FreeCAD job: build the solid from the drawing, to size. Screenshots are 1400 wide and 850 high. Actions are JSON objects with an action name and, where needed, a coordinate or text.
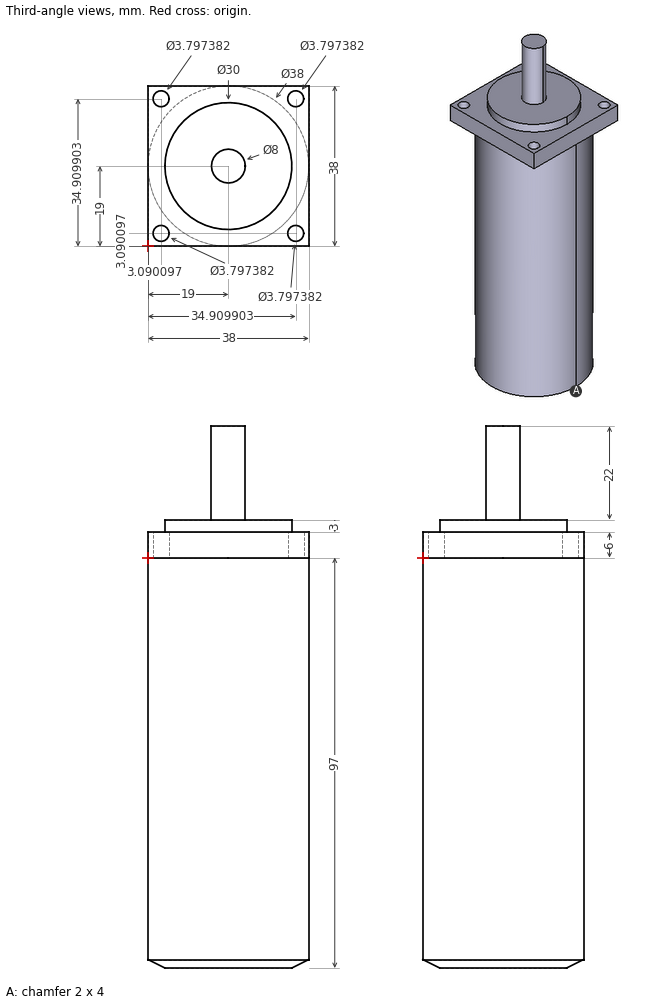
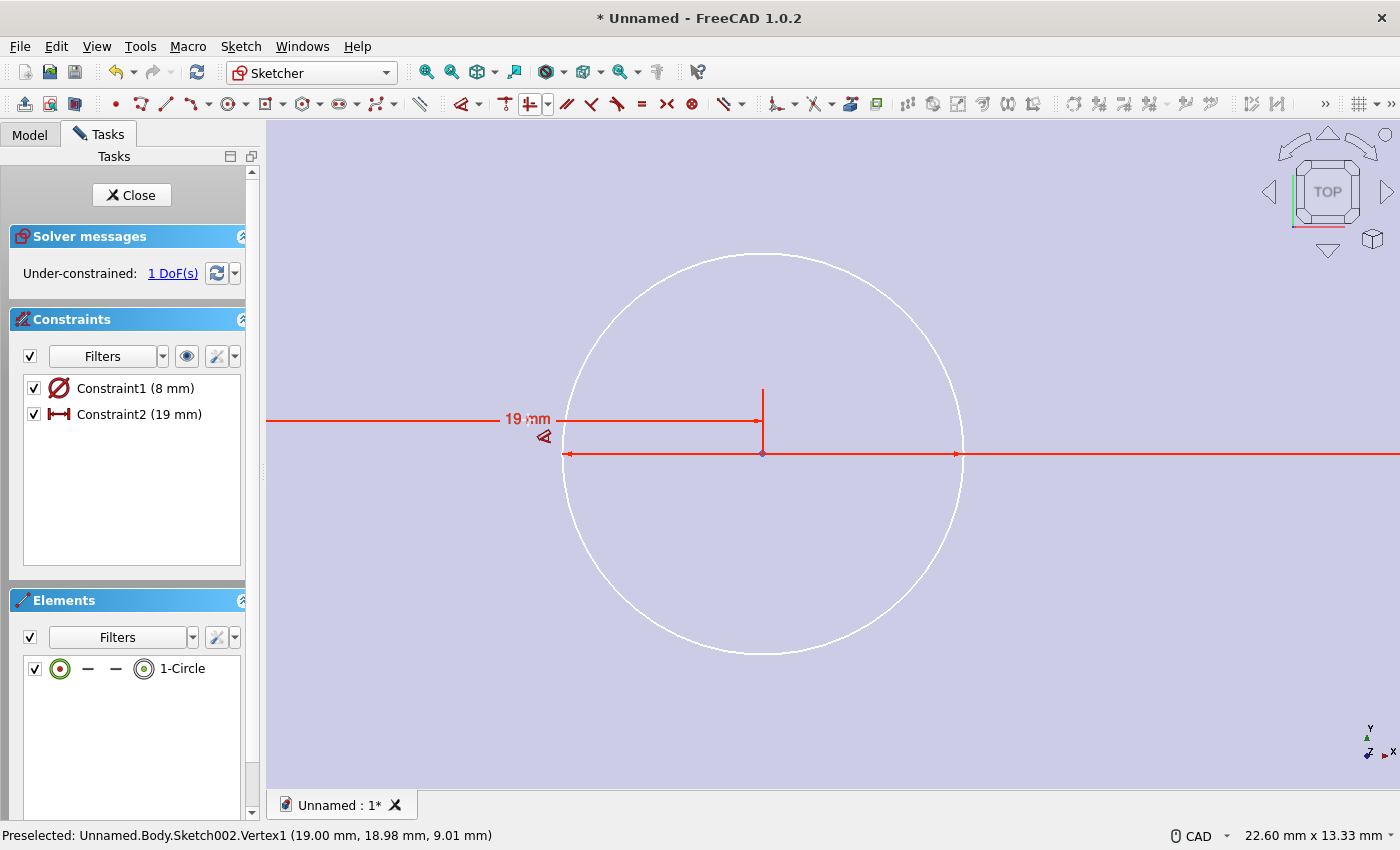
{"action": "left_click", "coordinate": [763, 454]}
{"action": "left_click", "coordinate": [797, 608]}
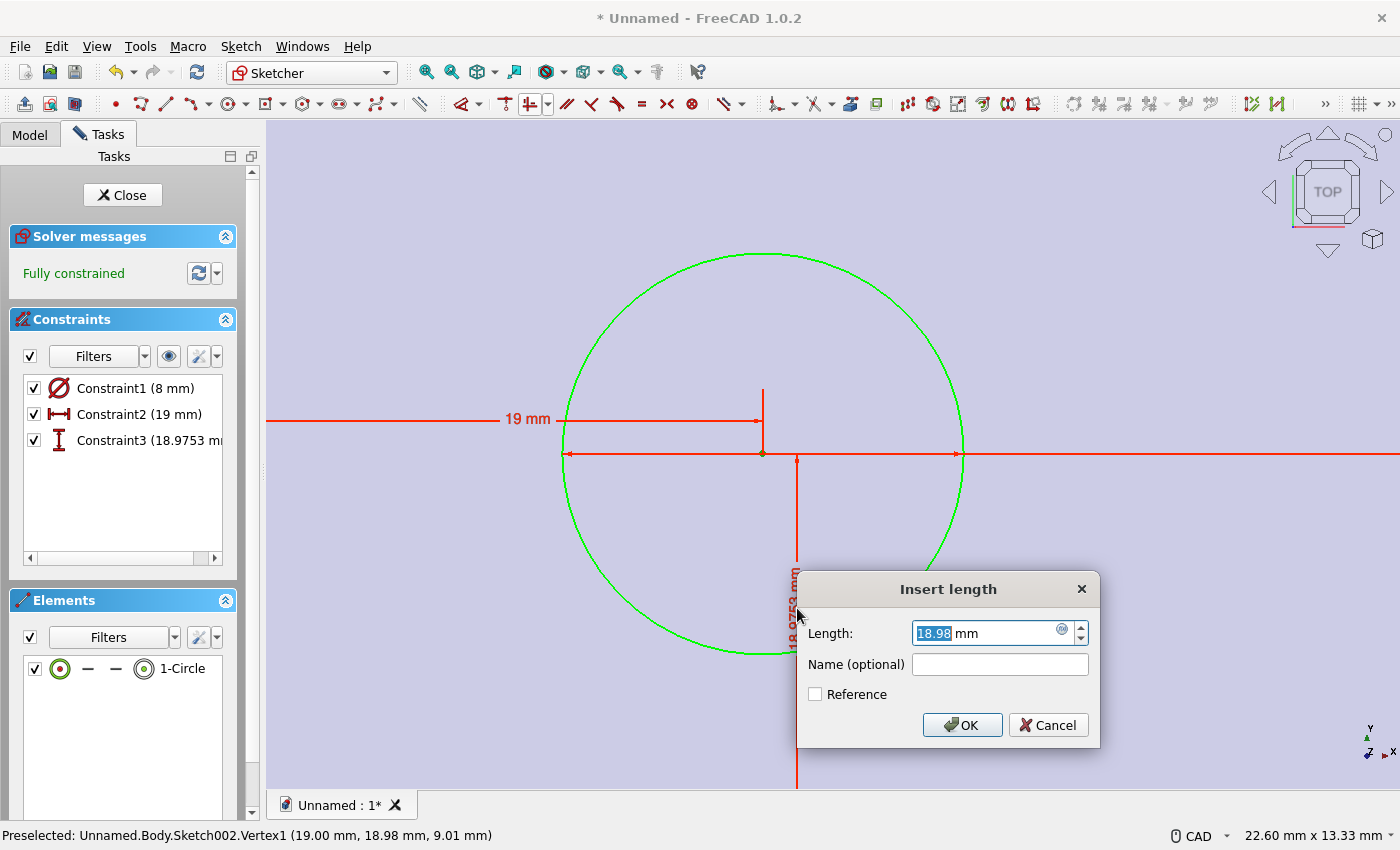
{"action": "type", "text": "19"}
{"action": "key", "text": "Return"}
{"action": "key", "text": "Escape"}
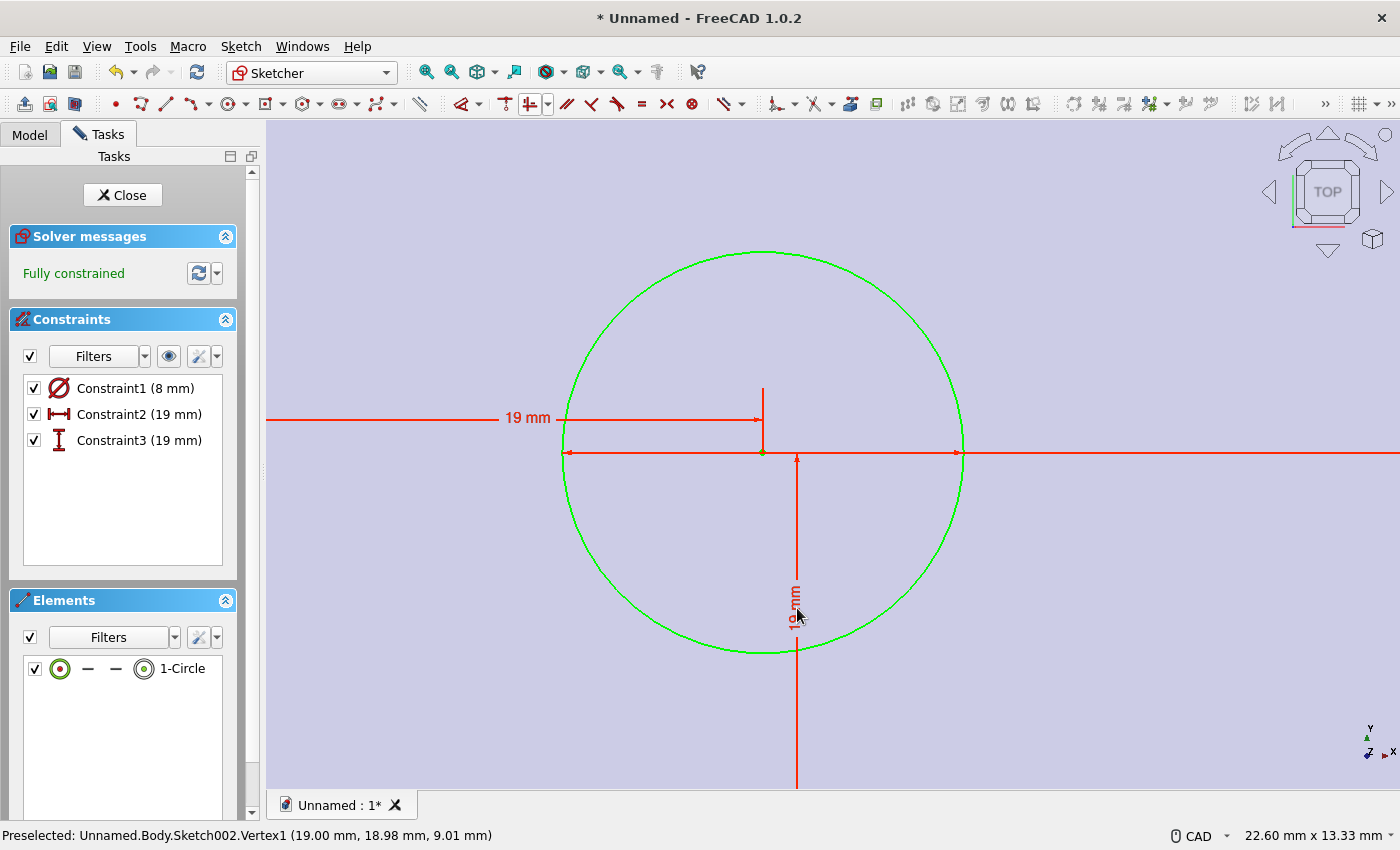
{"action": "left_click", "coordinate": [123, 195]}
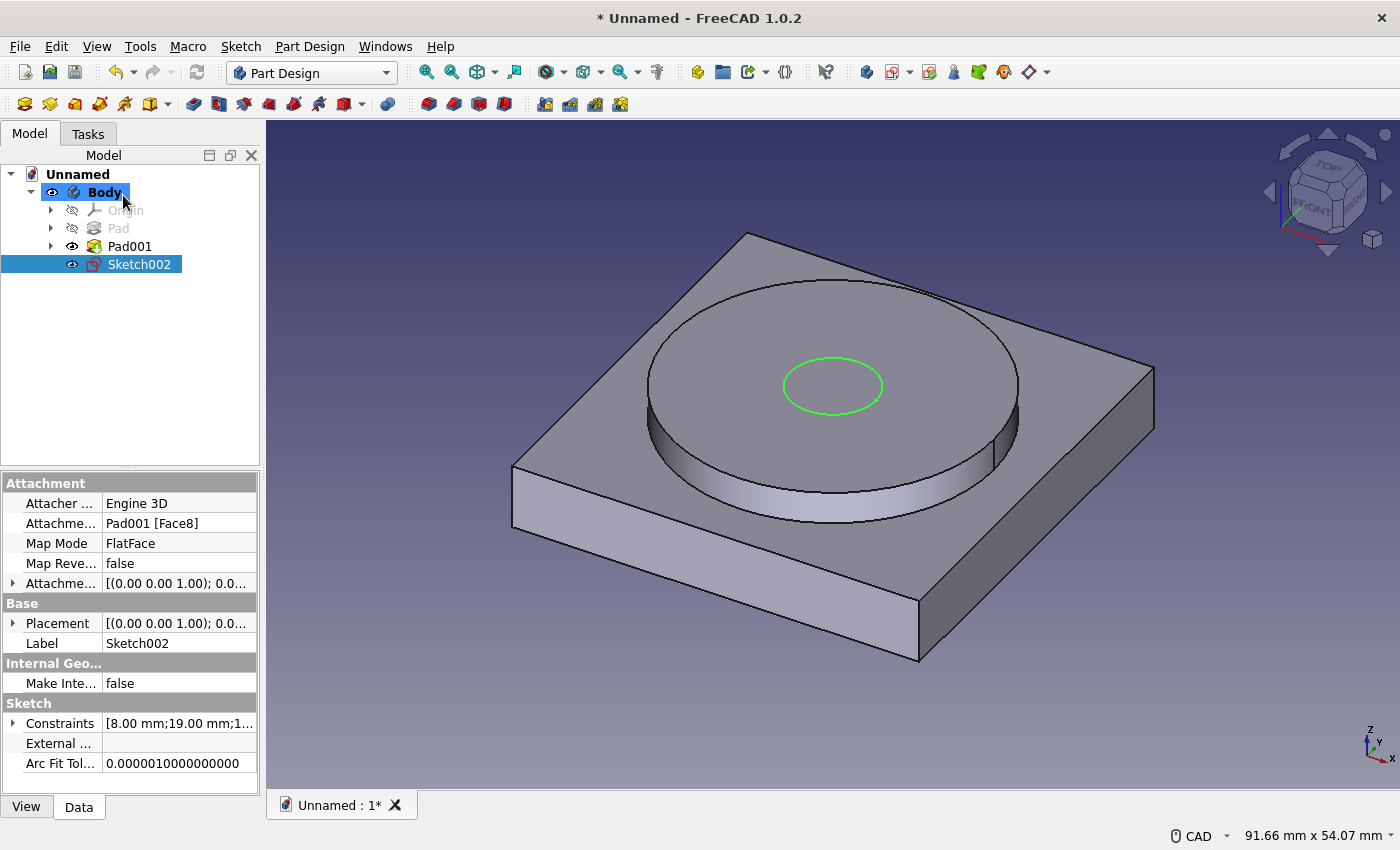
{"action": "left_click", "coordinate": [25, 104]}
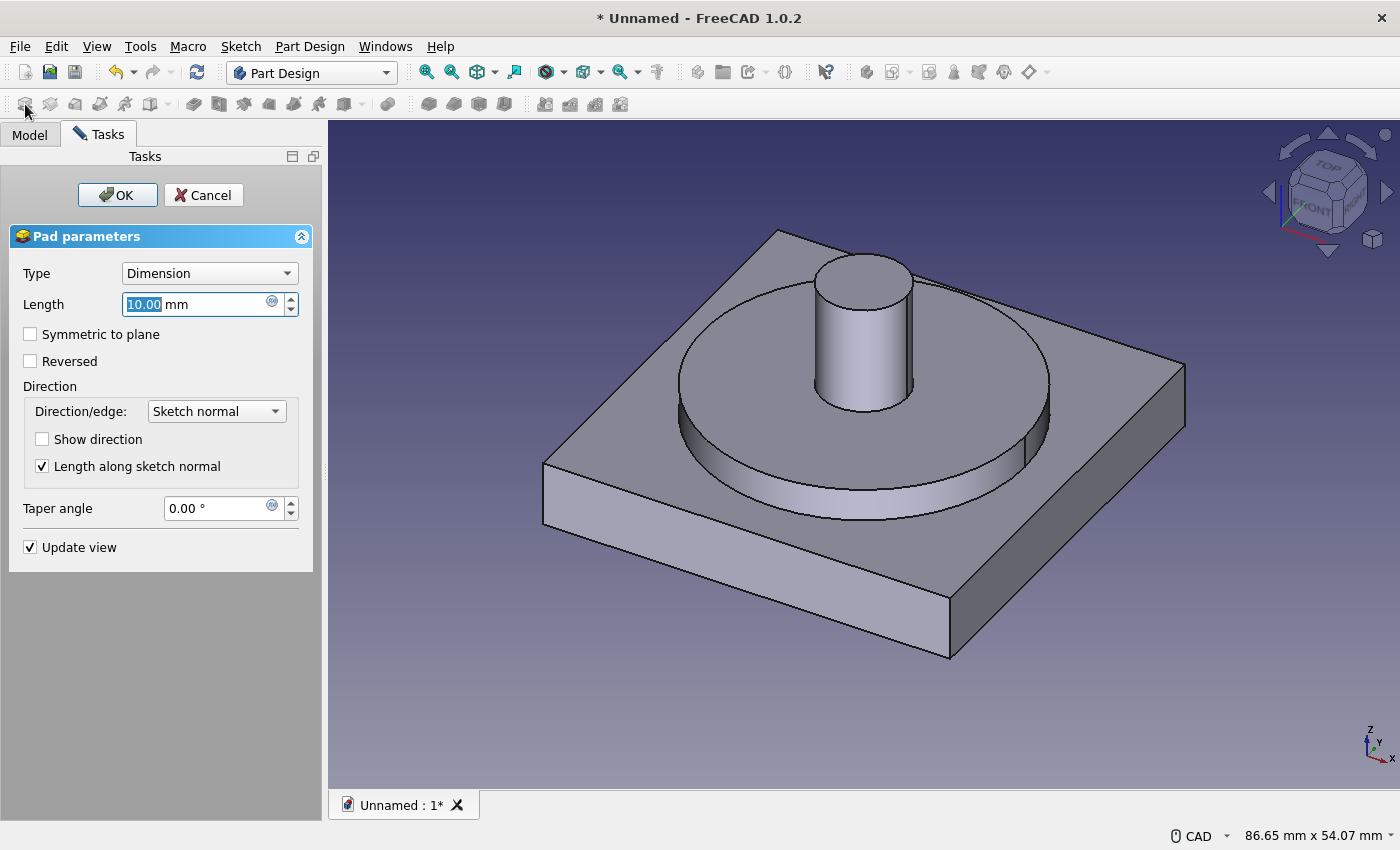
{"action": "type", "text": "22"}
{"action": "key", "text": "Tab"}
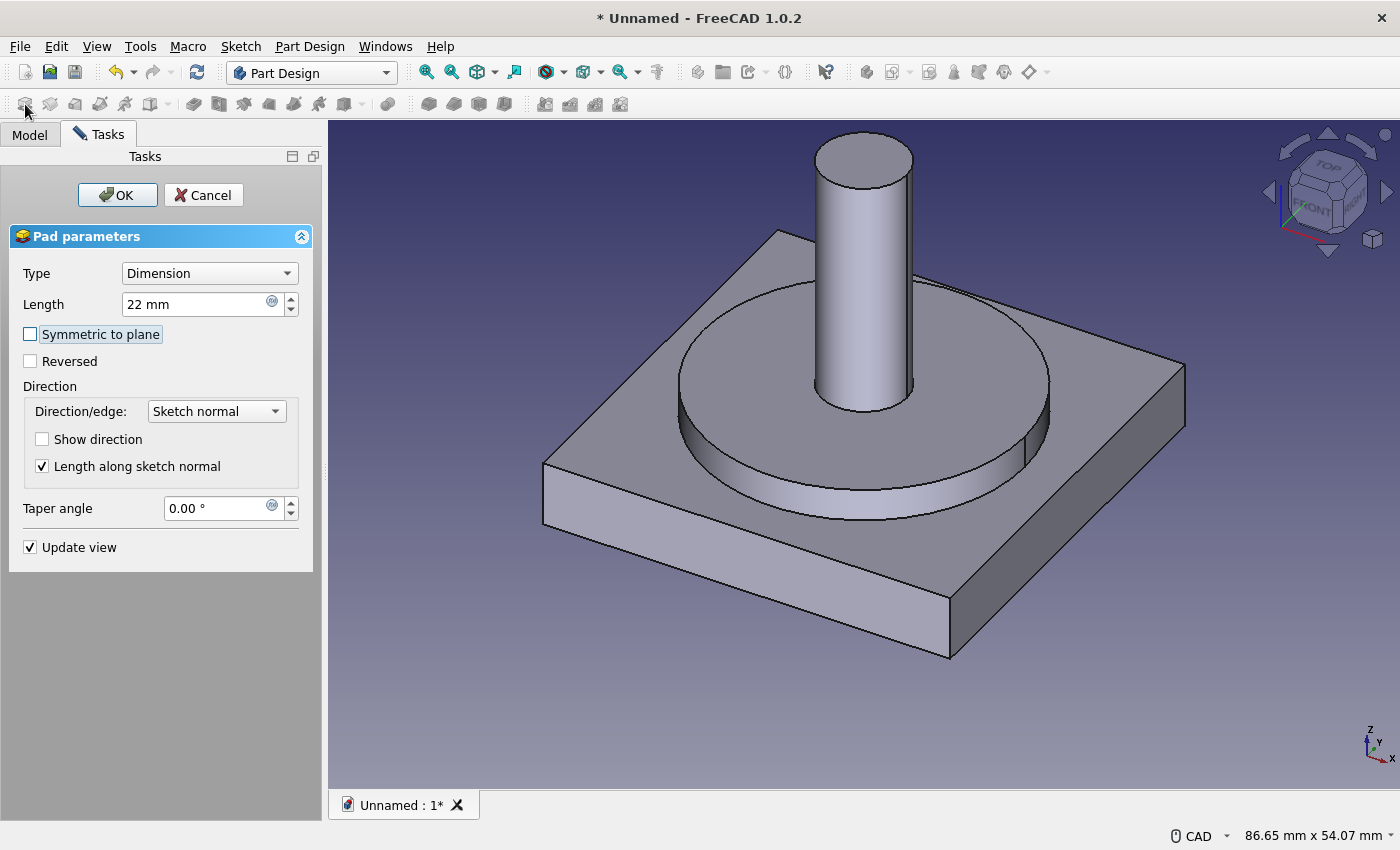
{"action": "left_click", "coordinate": [118, 195]}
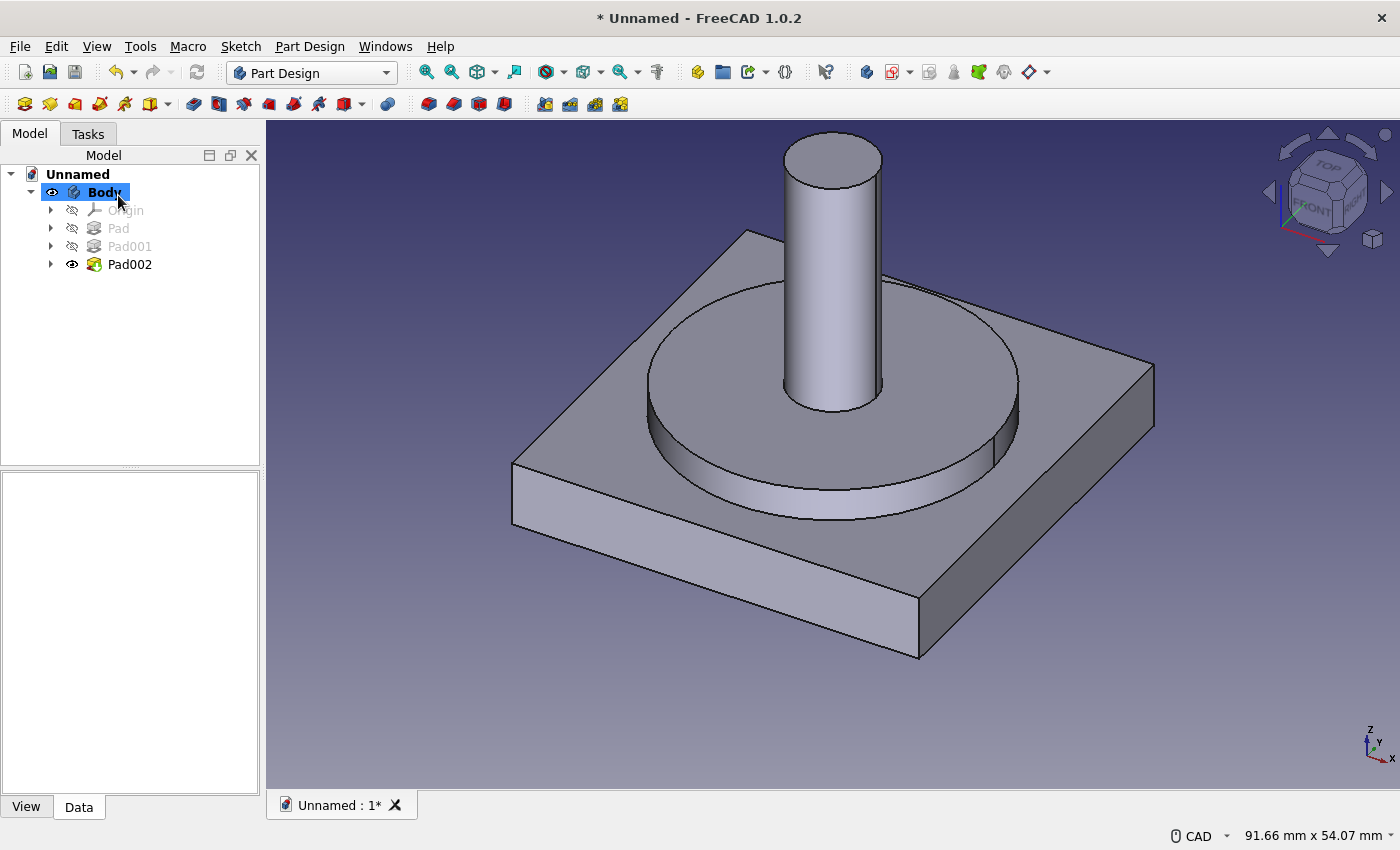
{"action": "key", "text": "v f"}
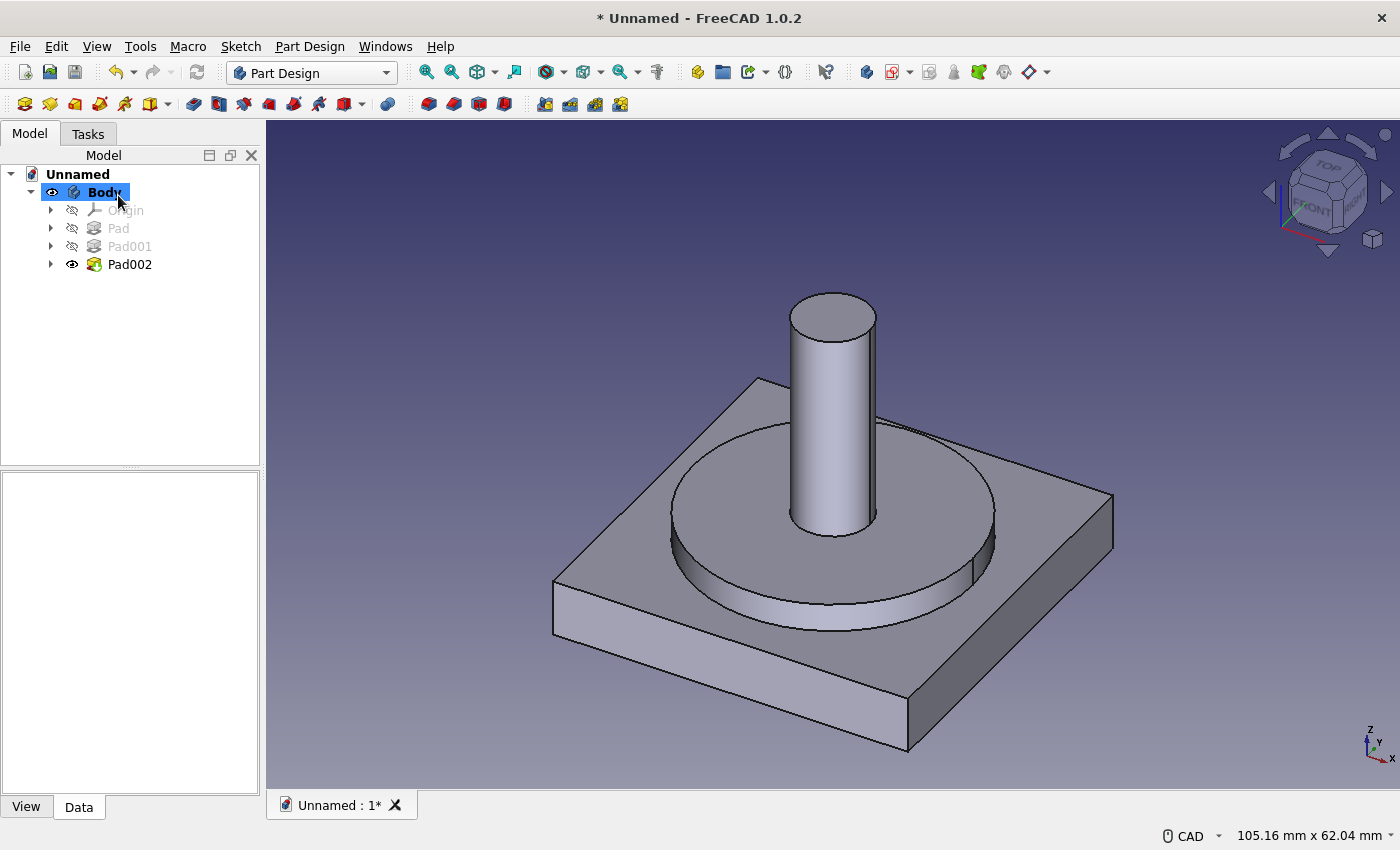
{"action": "key", "text": "5"}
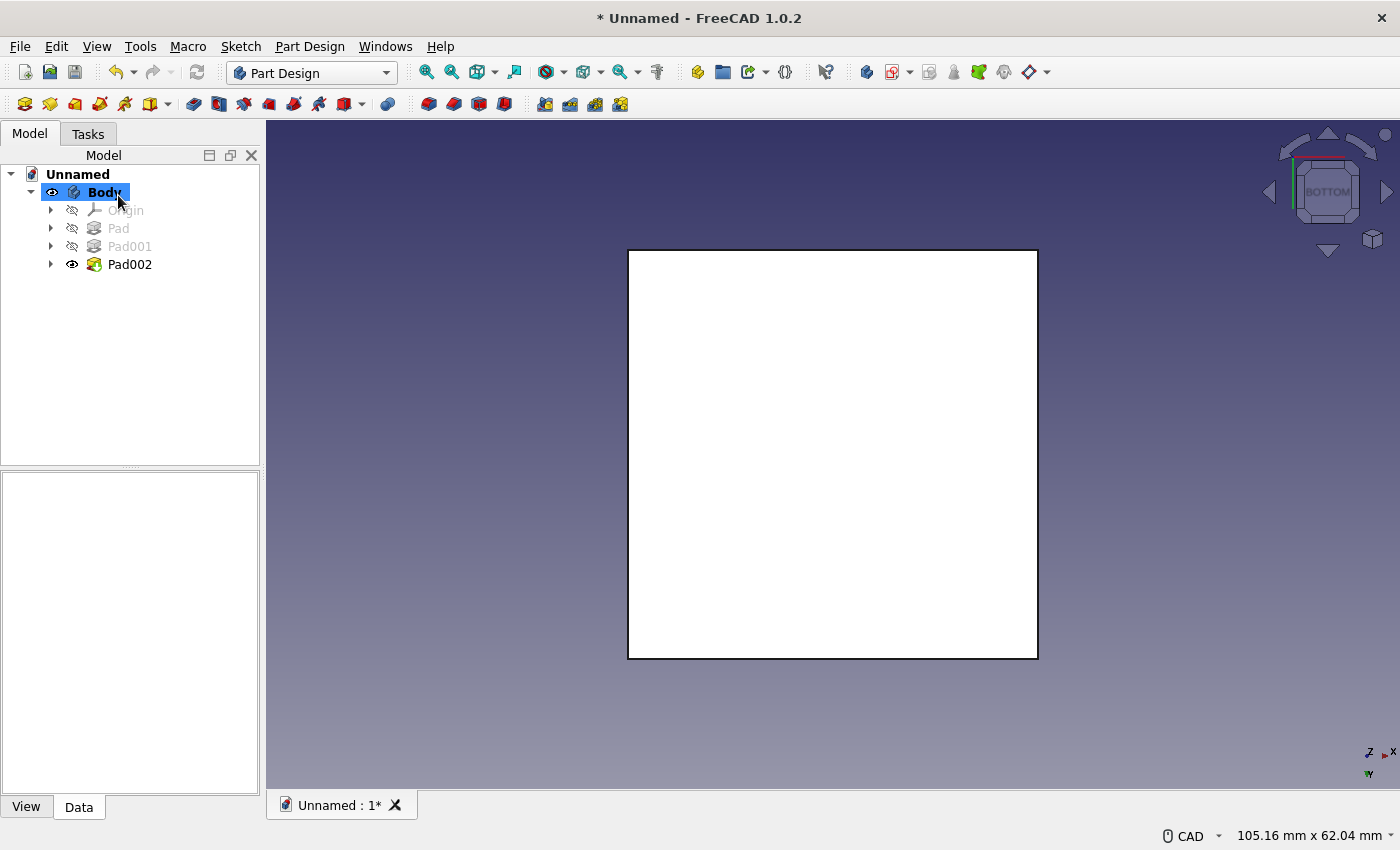
{"action": "left_click", "coordinate": [833, 453]}